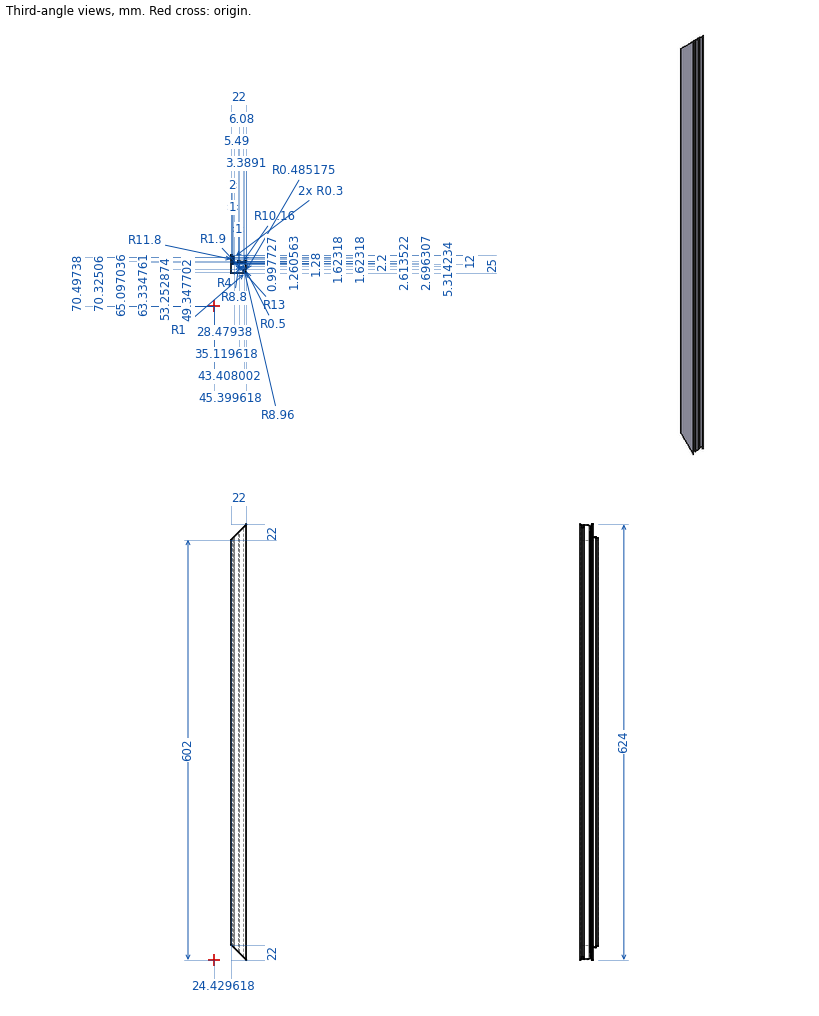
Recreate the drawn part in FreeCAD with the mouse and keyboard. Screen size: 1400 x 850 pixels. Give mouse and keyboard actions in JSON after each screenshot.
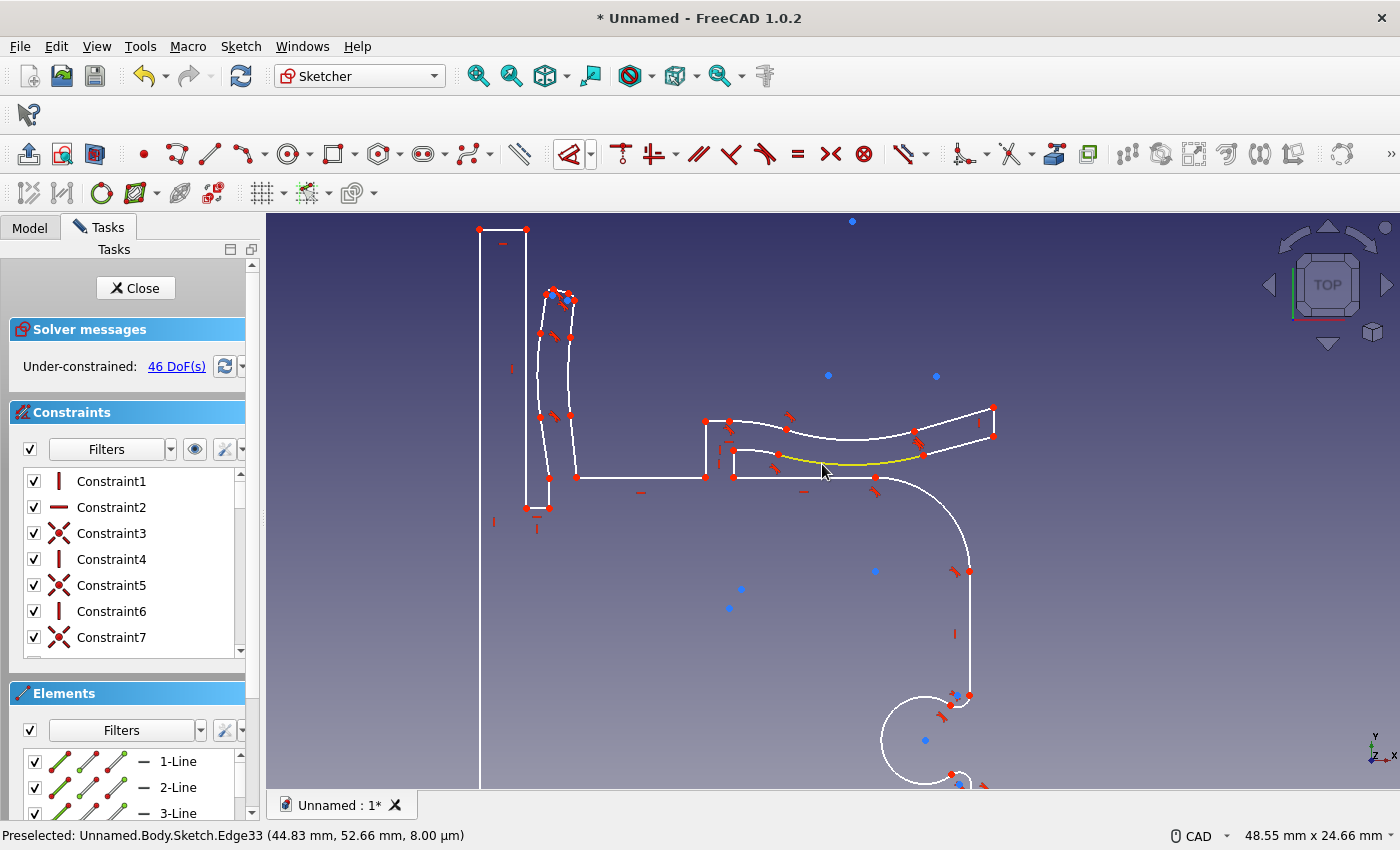
{"action": "left_click", "coordinate": [822, 463]}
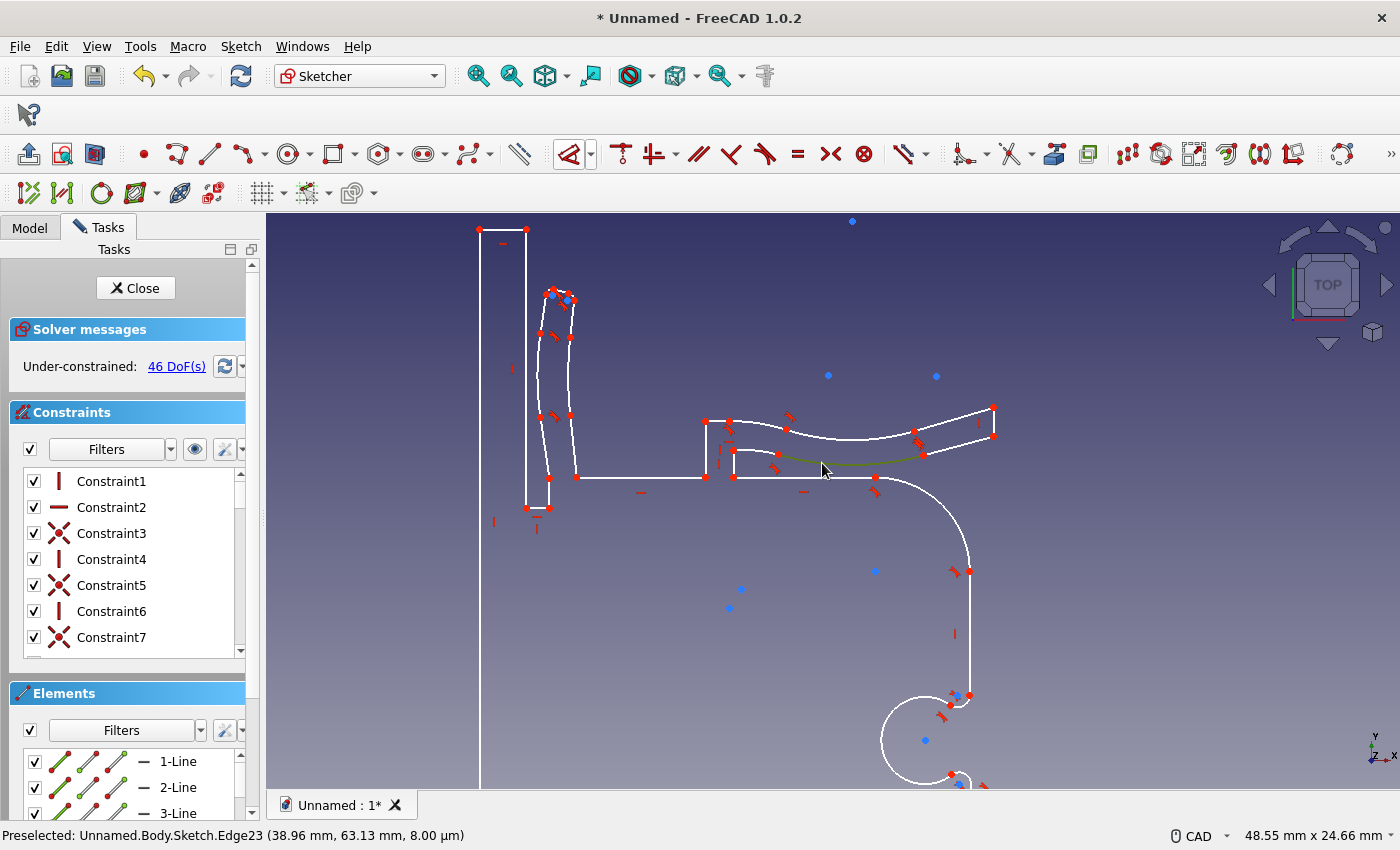
{"action": "left_click", "coordinate": [824, 438]}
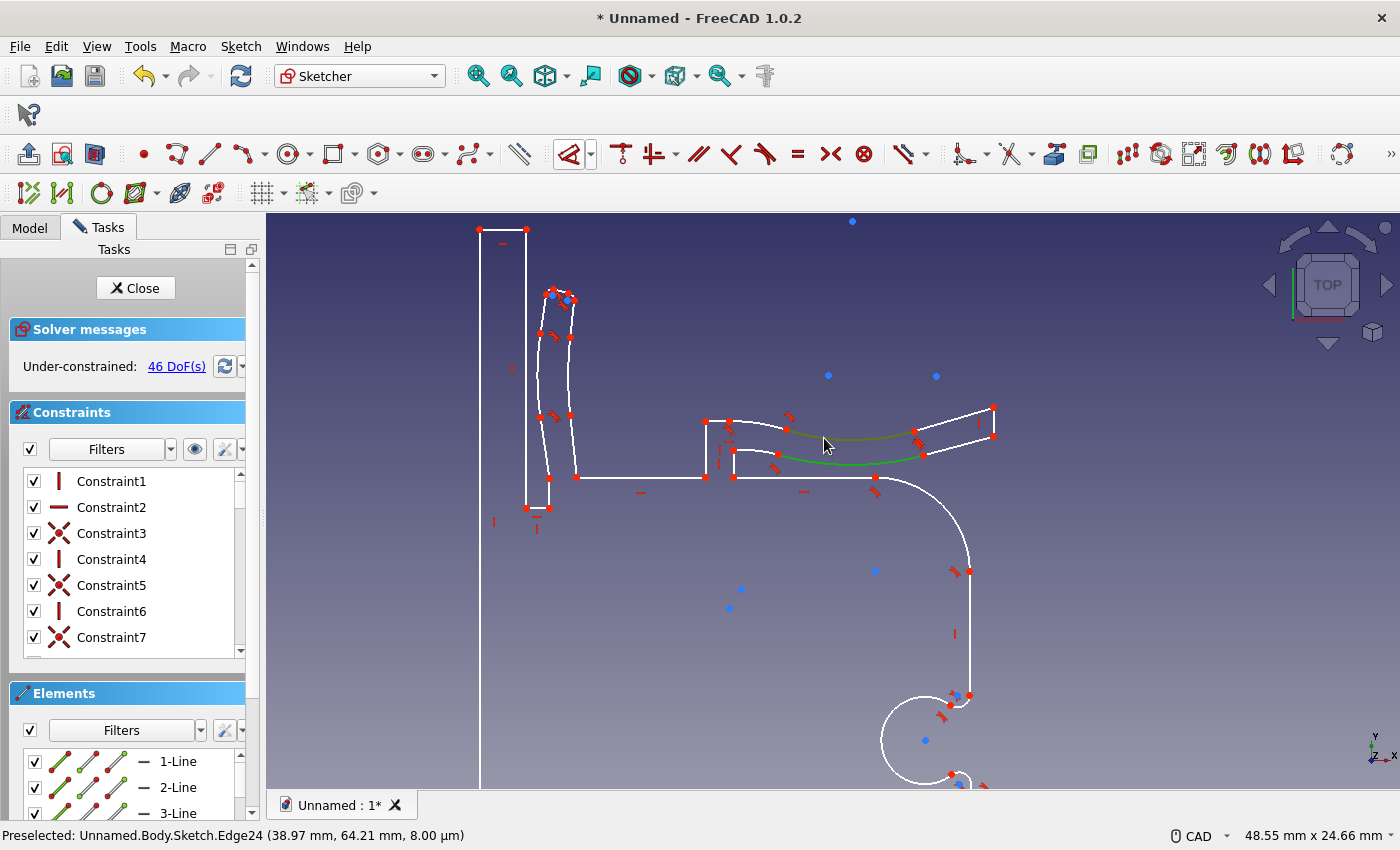
{"action": "key", "text": "c"}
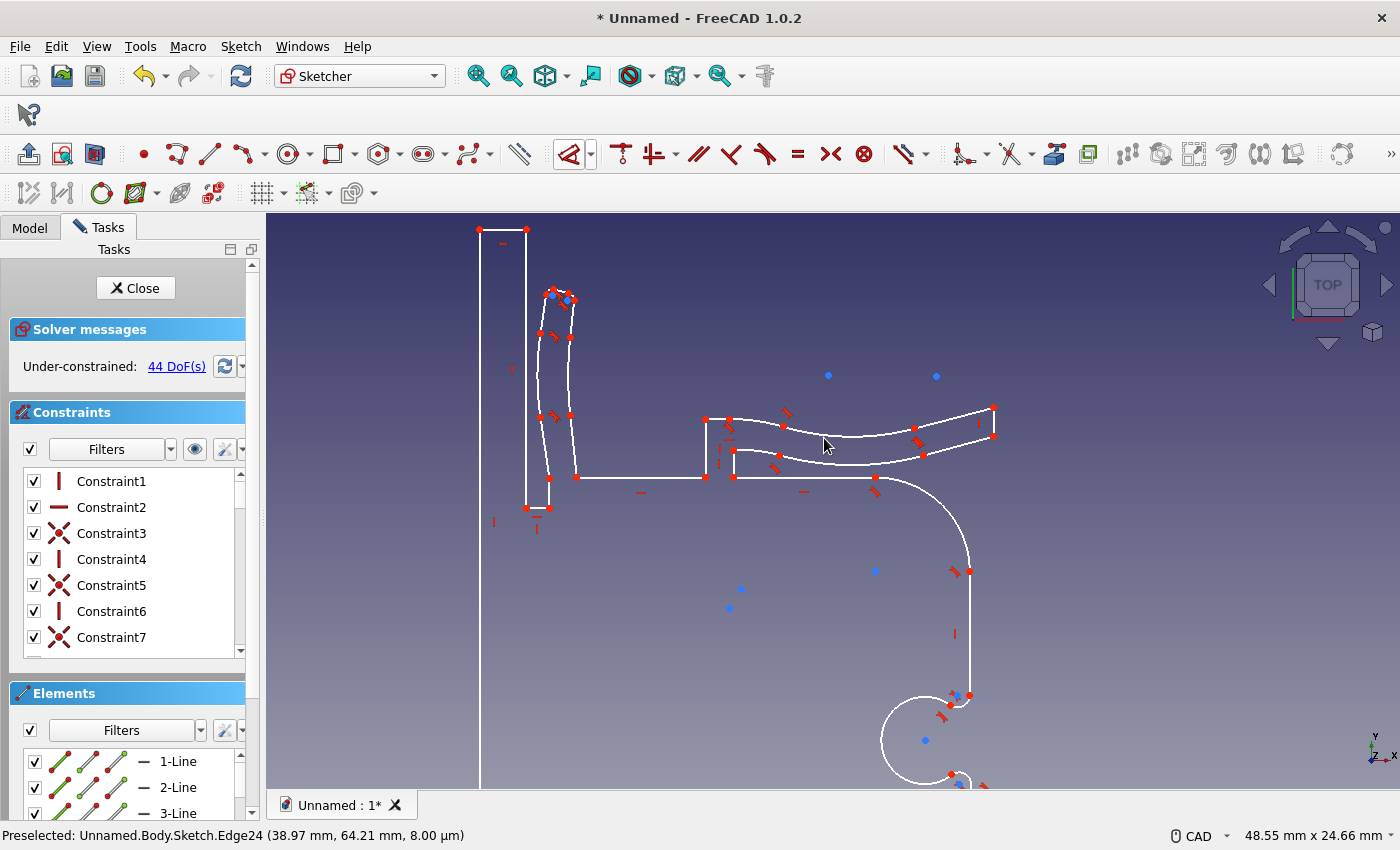
{"action": "left_click", "coordinate": [766, 452]}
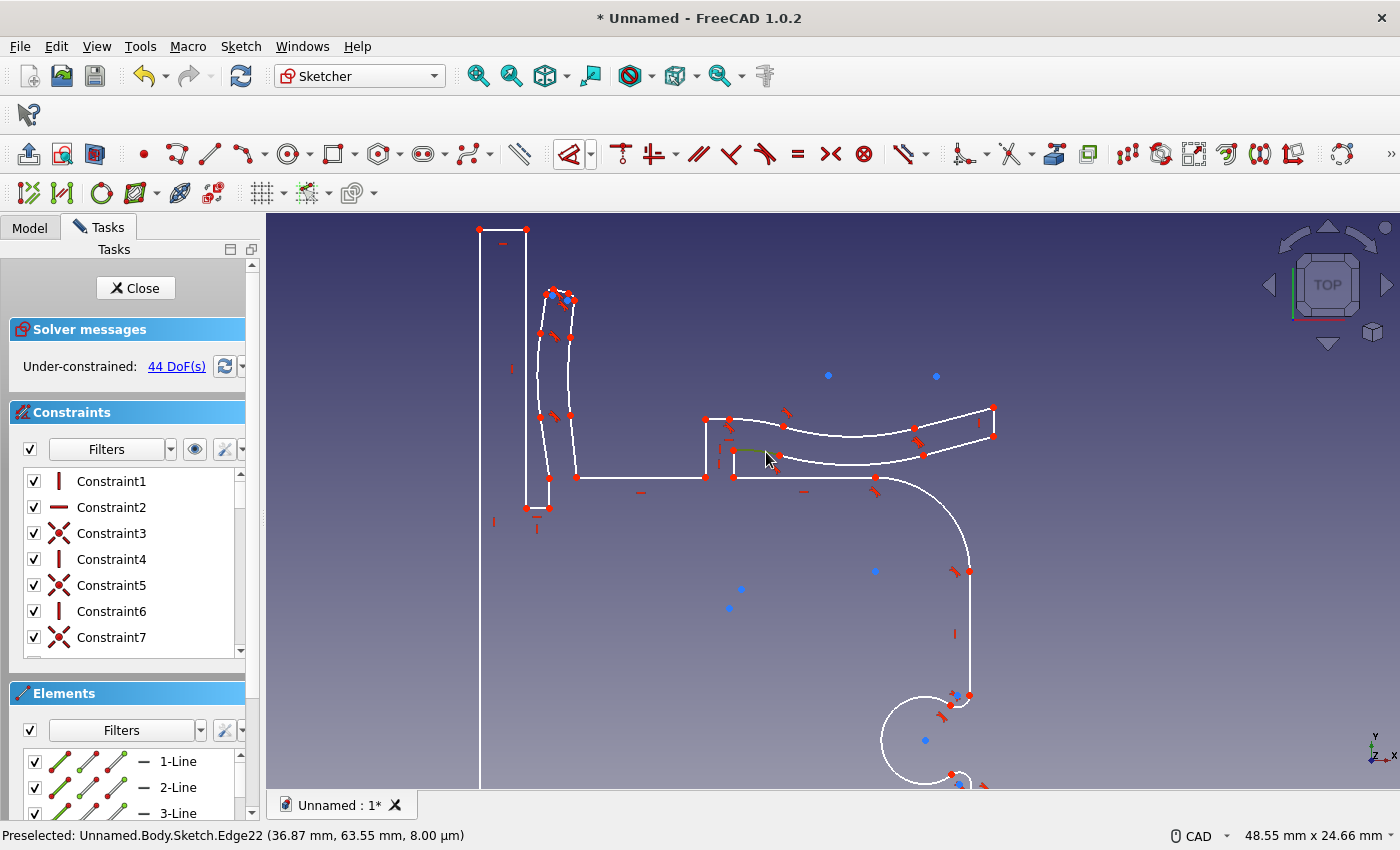
{"action": "left_click", "coordinate": [767, 423]}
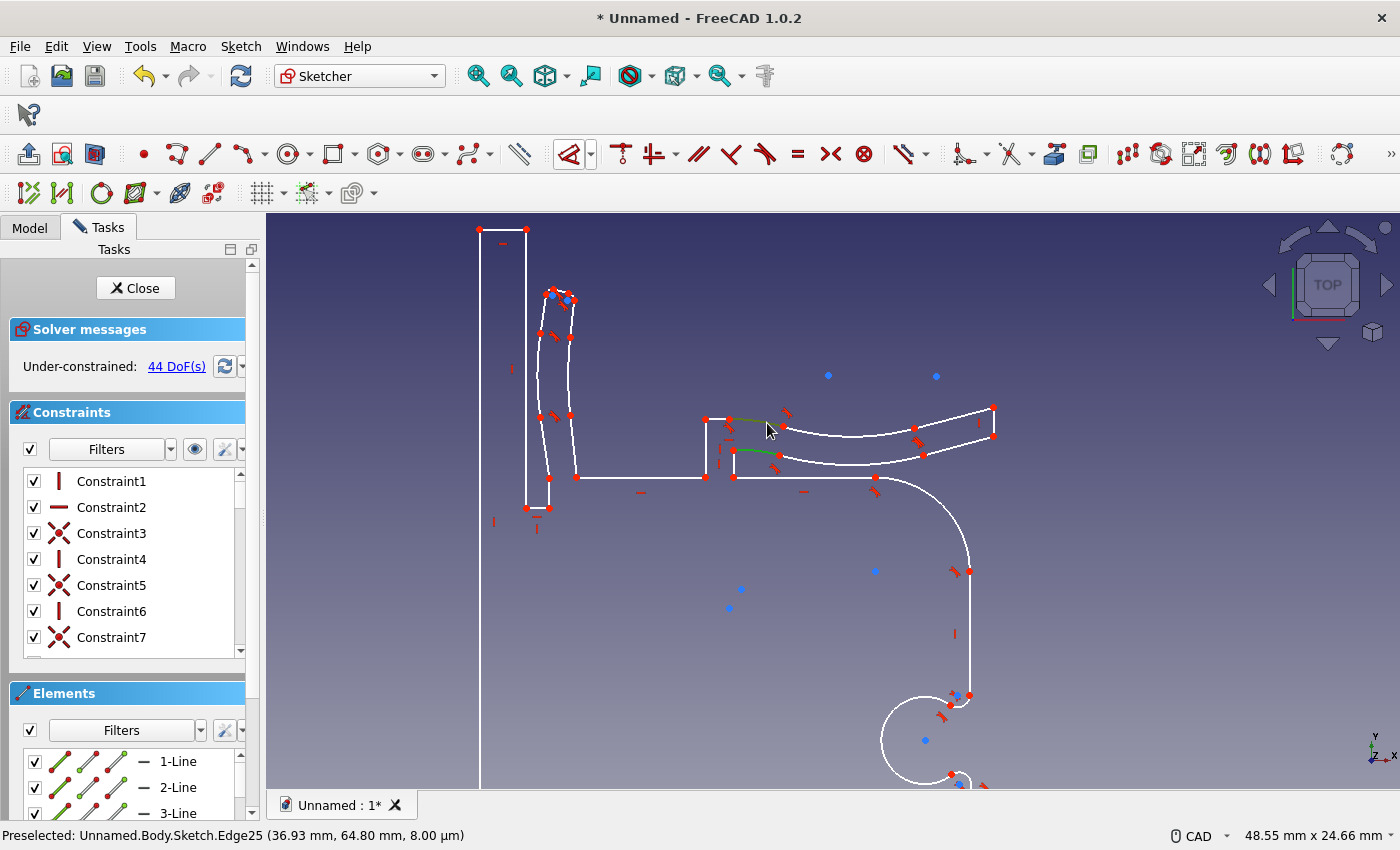
{"action": "key", "text": "c"}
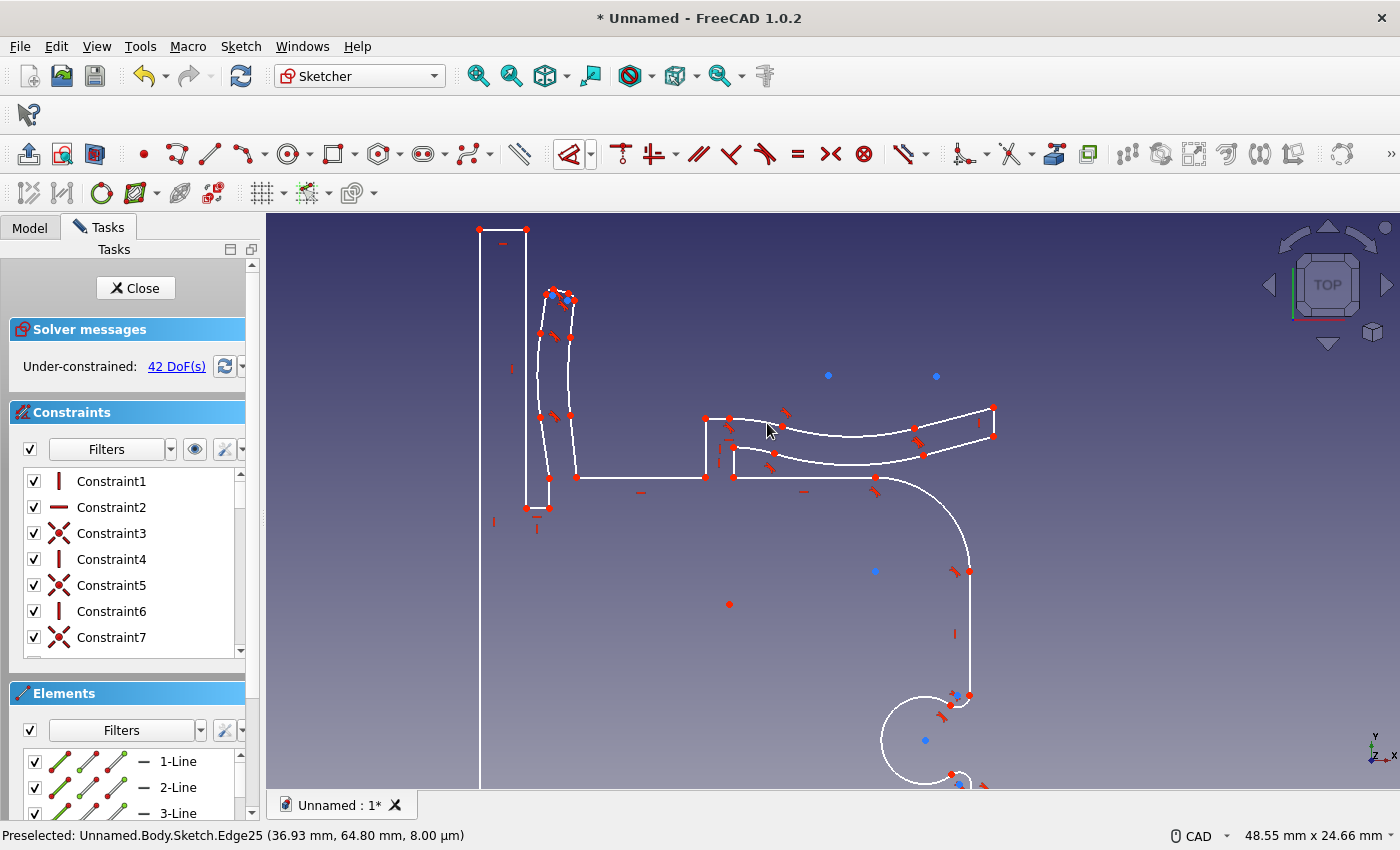
{"action": "left_click", "coordinate": [569, 361]}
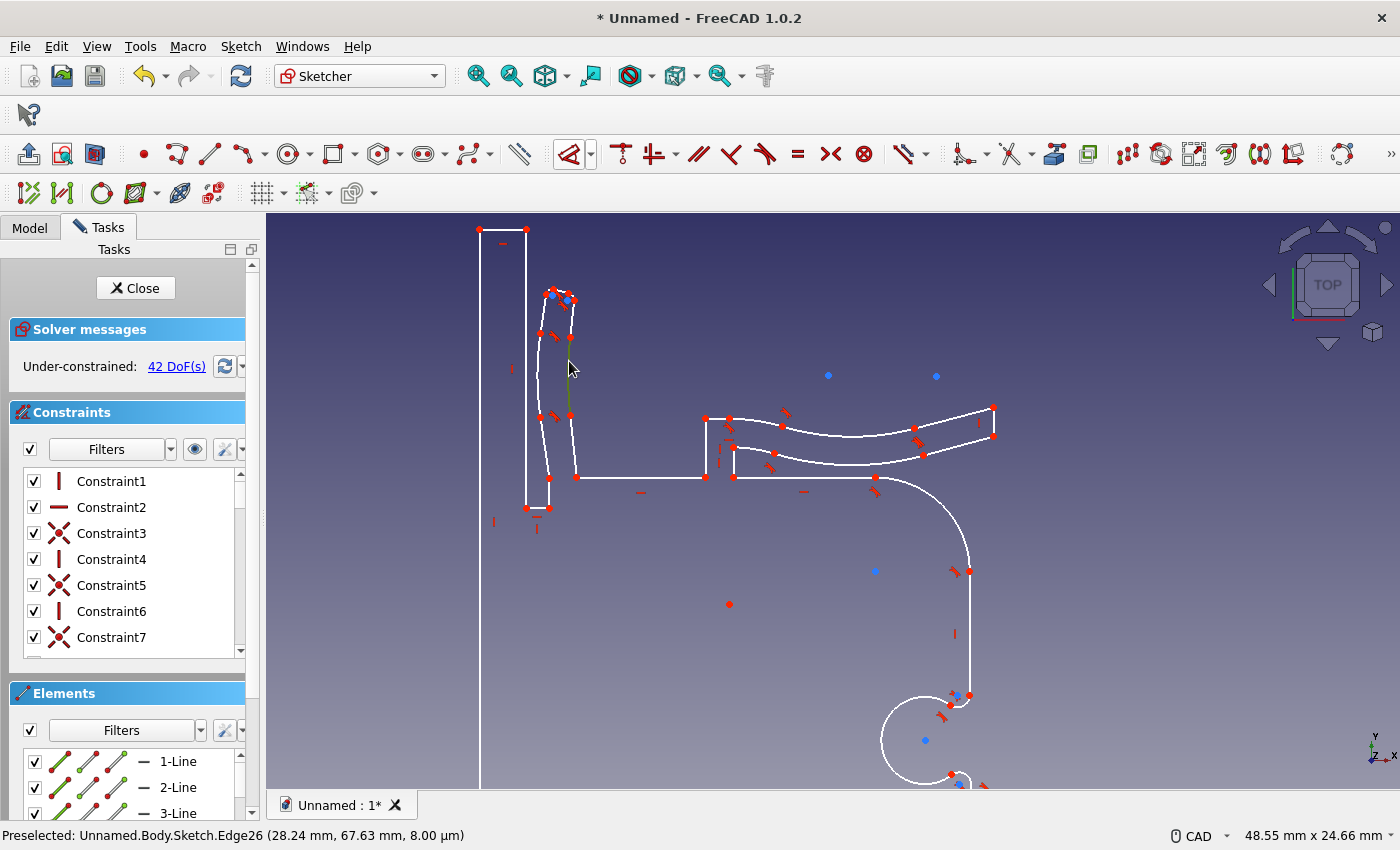
{"action": "left_click", "coordinate": [538, 358]}